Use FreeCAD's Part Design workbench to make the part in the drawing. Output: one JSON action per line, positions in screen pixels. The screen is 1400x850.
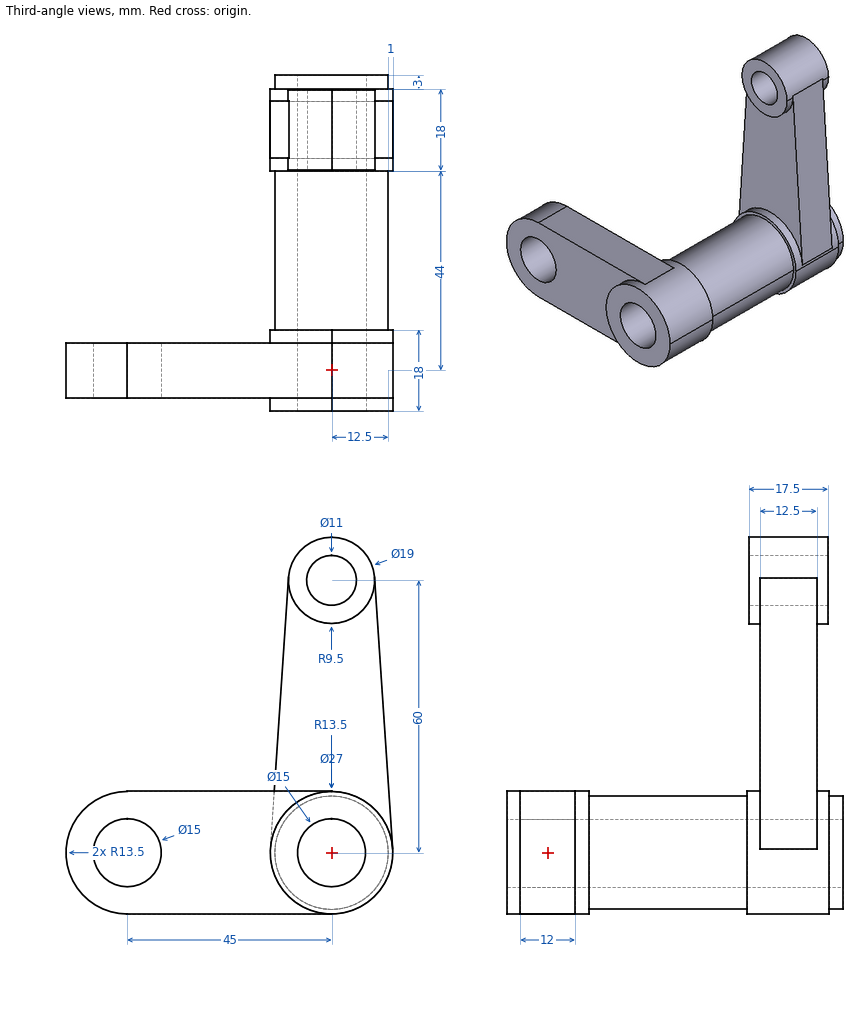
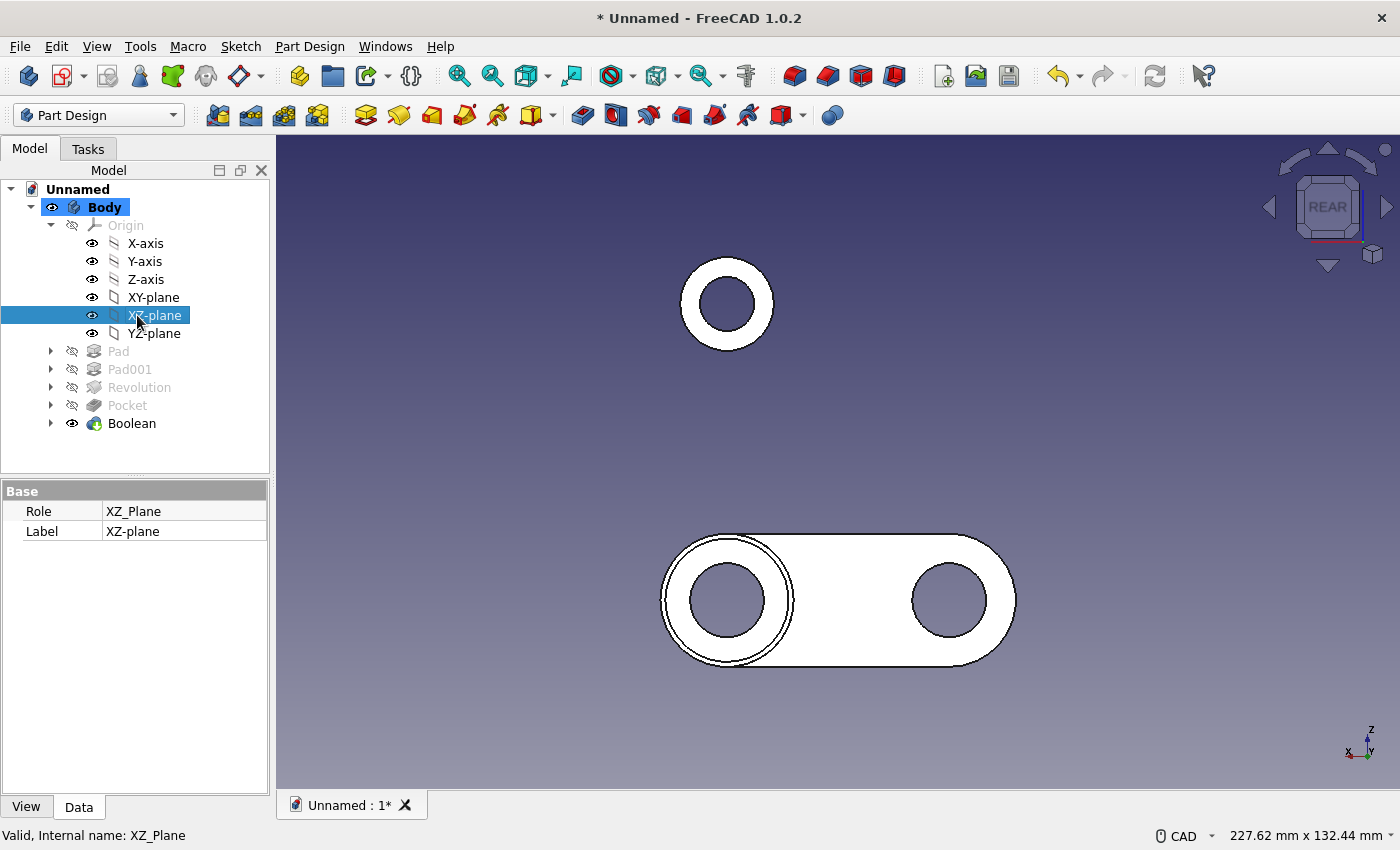
{"action": "left_click", "coordinate": [238, 76]}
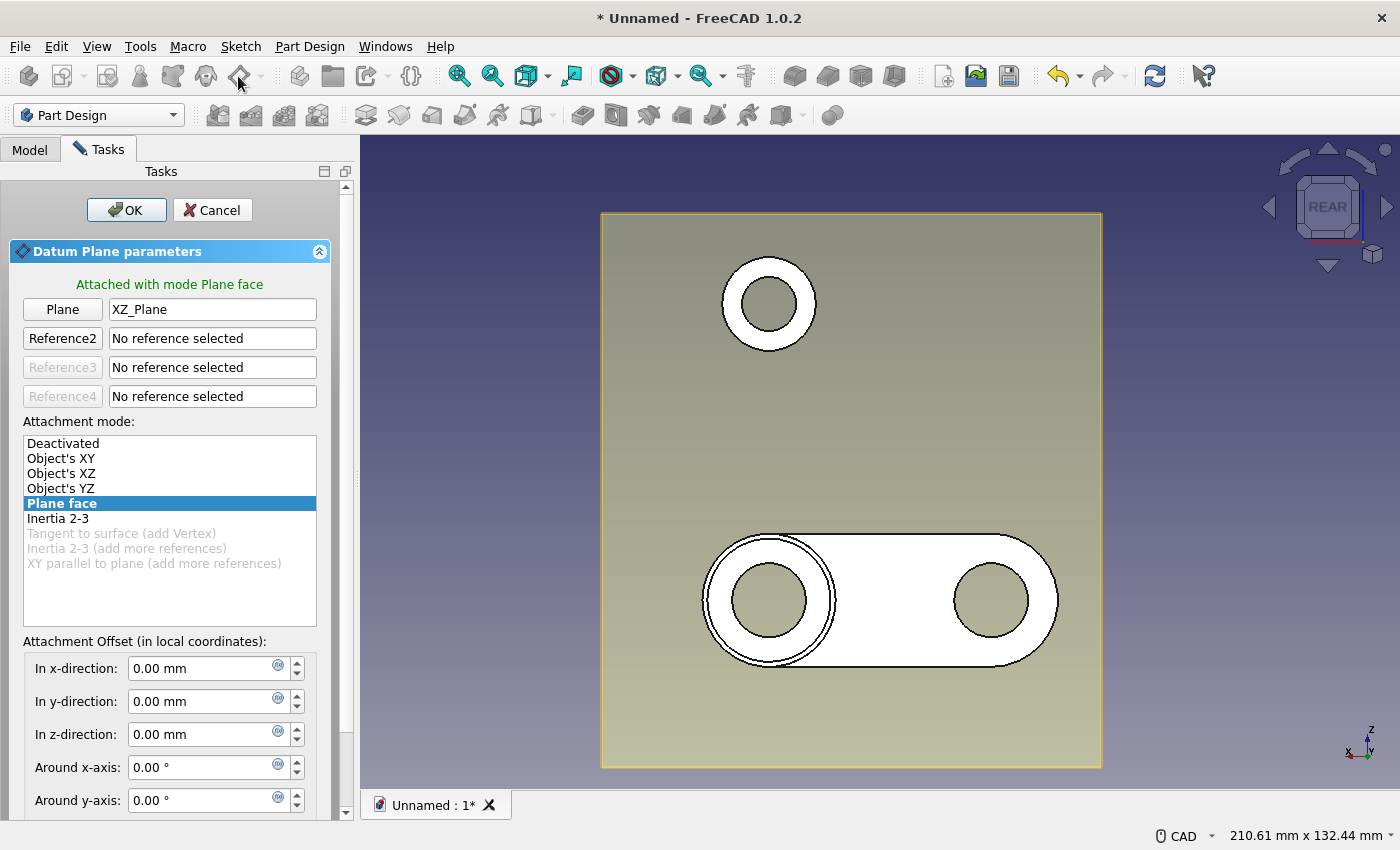
{"action": "triple_click", "coordinate": [210, 734]}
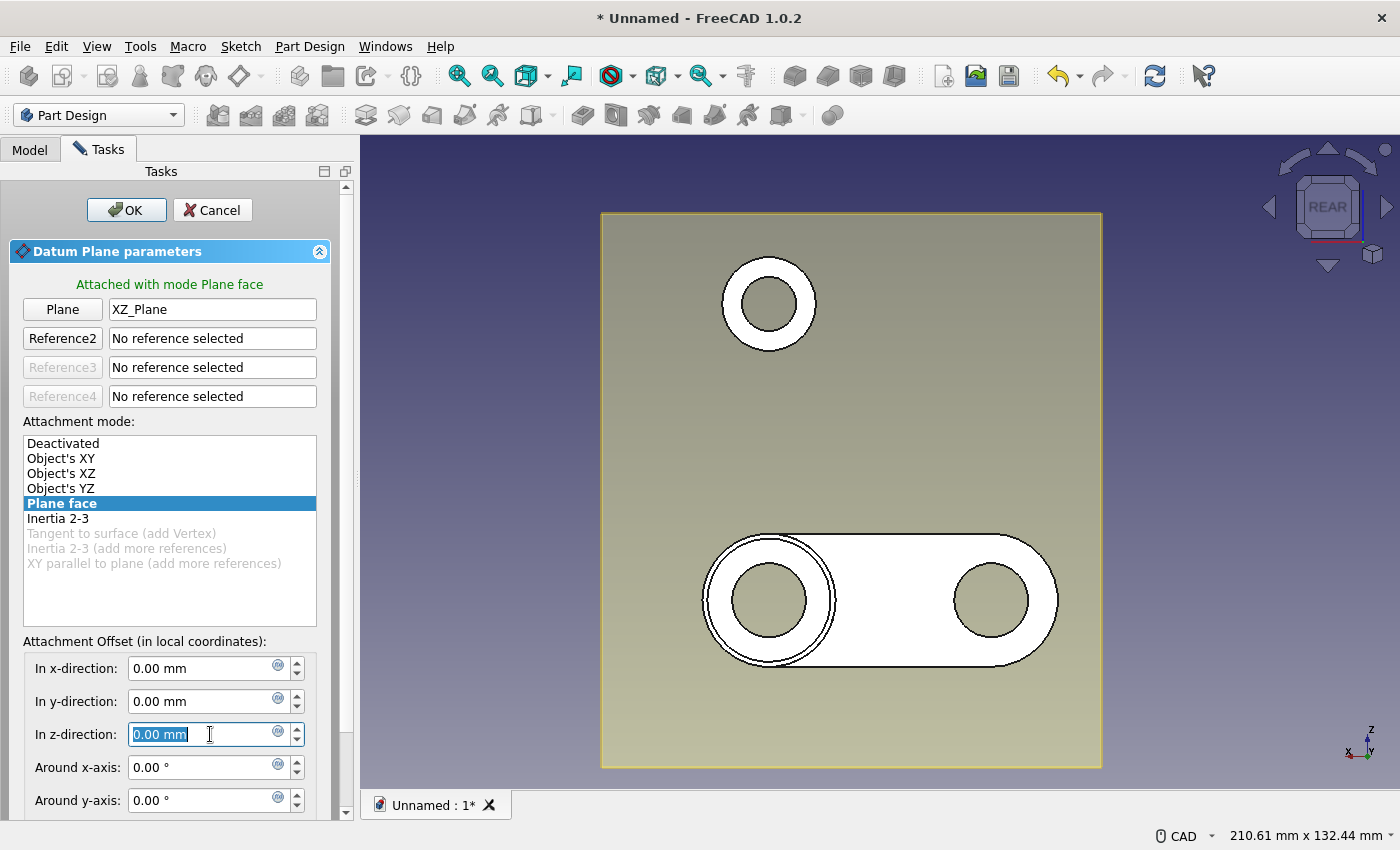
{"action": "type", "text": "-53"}
{"action": "key", "text": "Tab"}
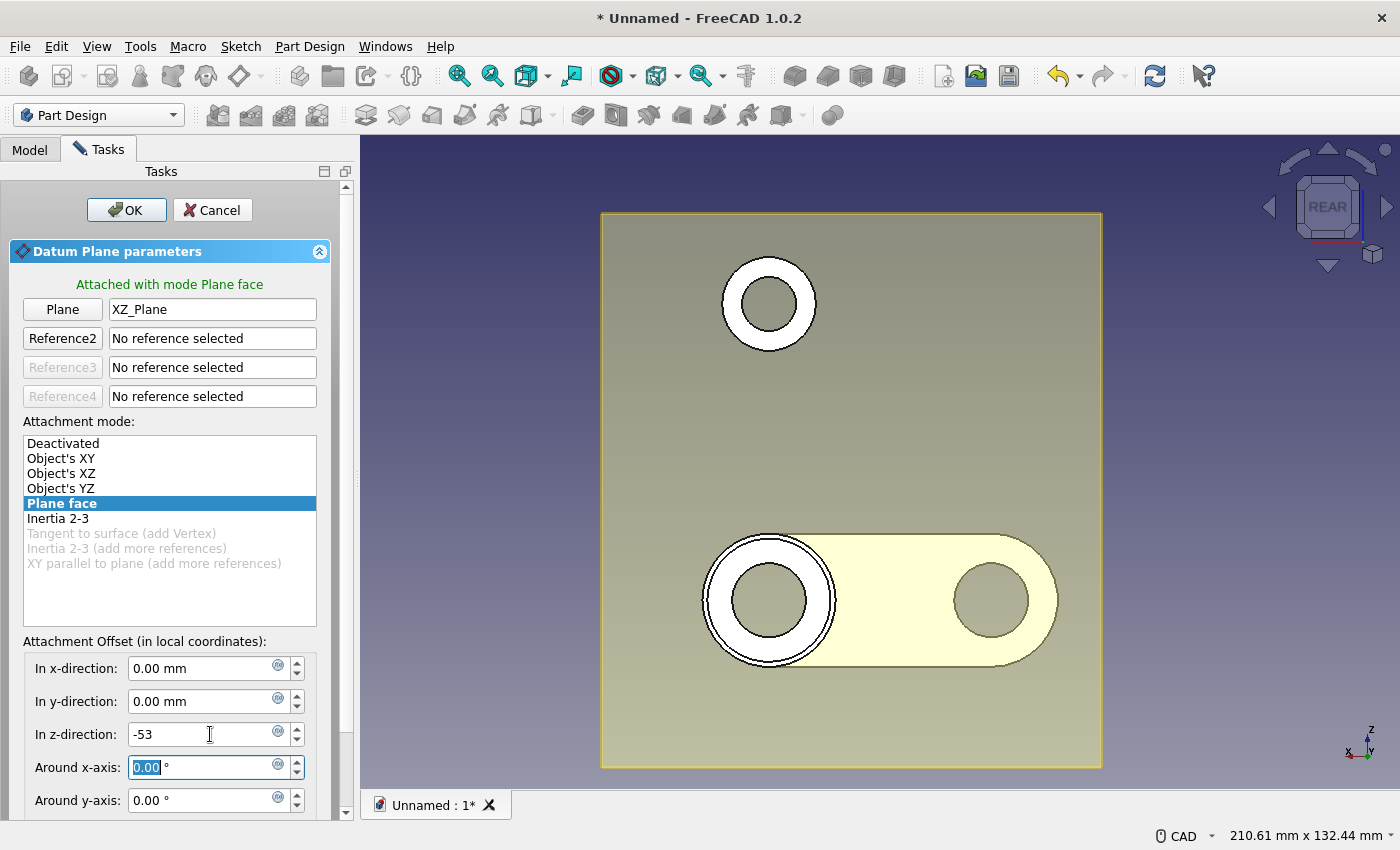
{"action": "left_click", "coordinate": [127, 210]}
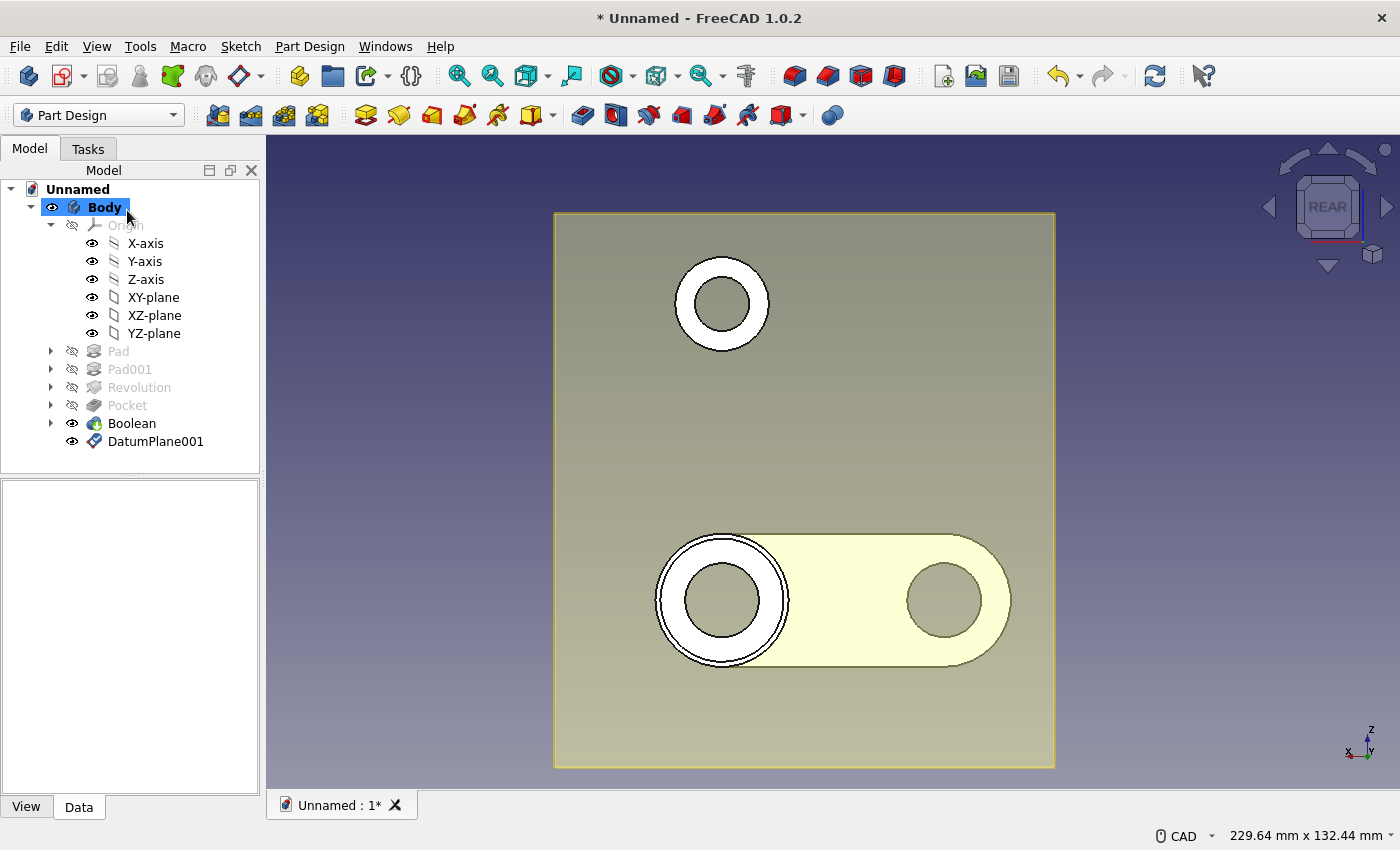
{"action": "left_click", "coordinate": [117, 441]}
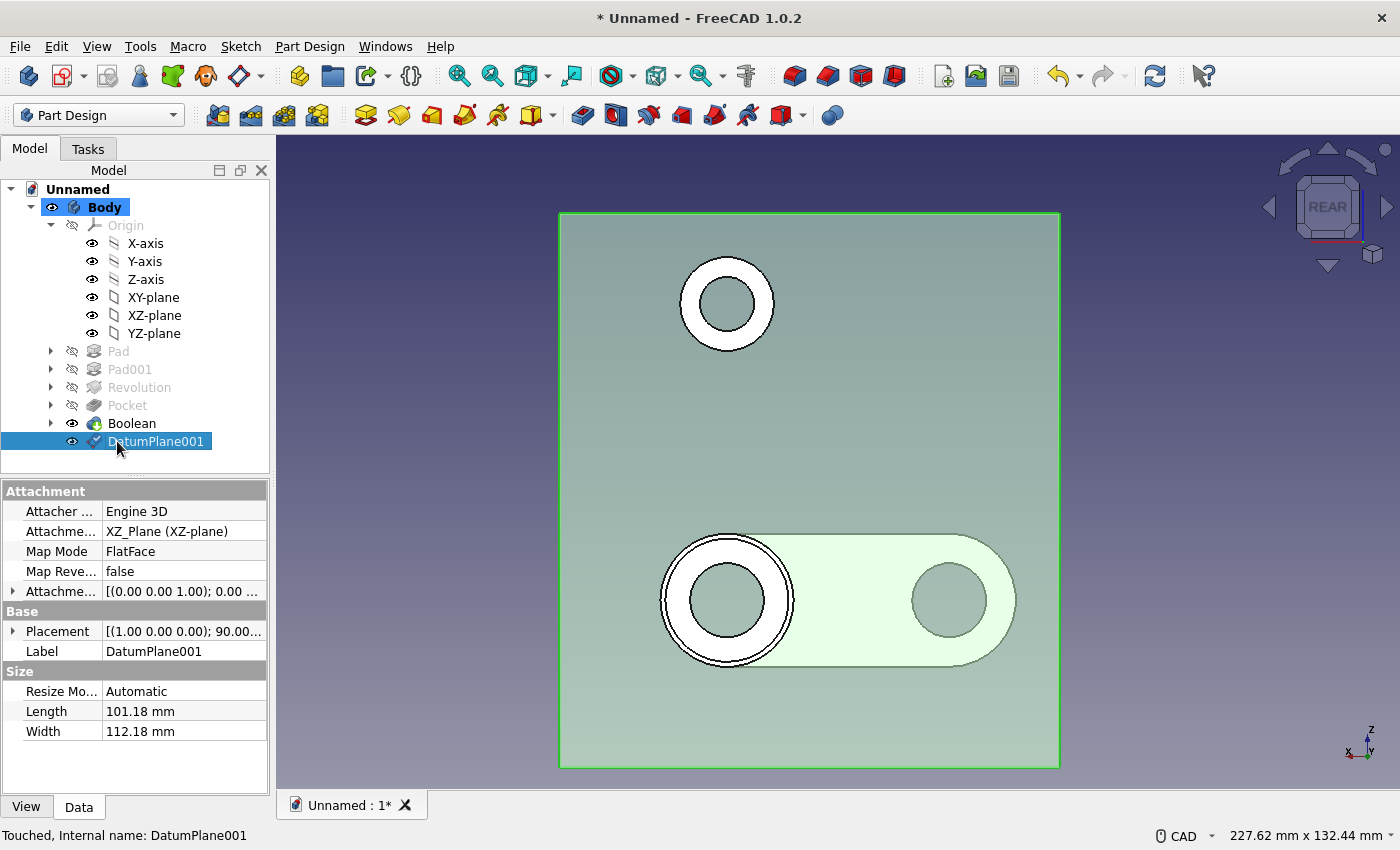
{"action": "left_click", "coordinate": [62, 76]}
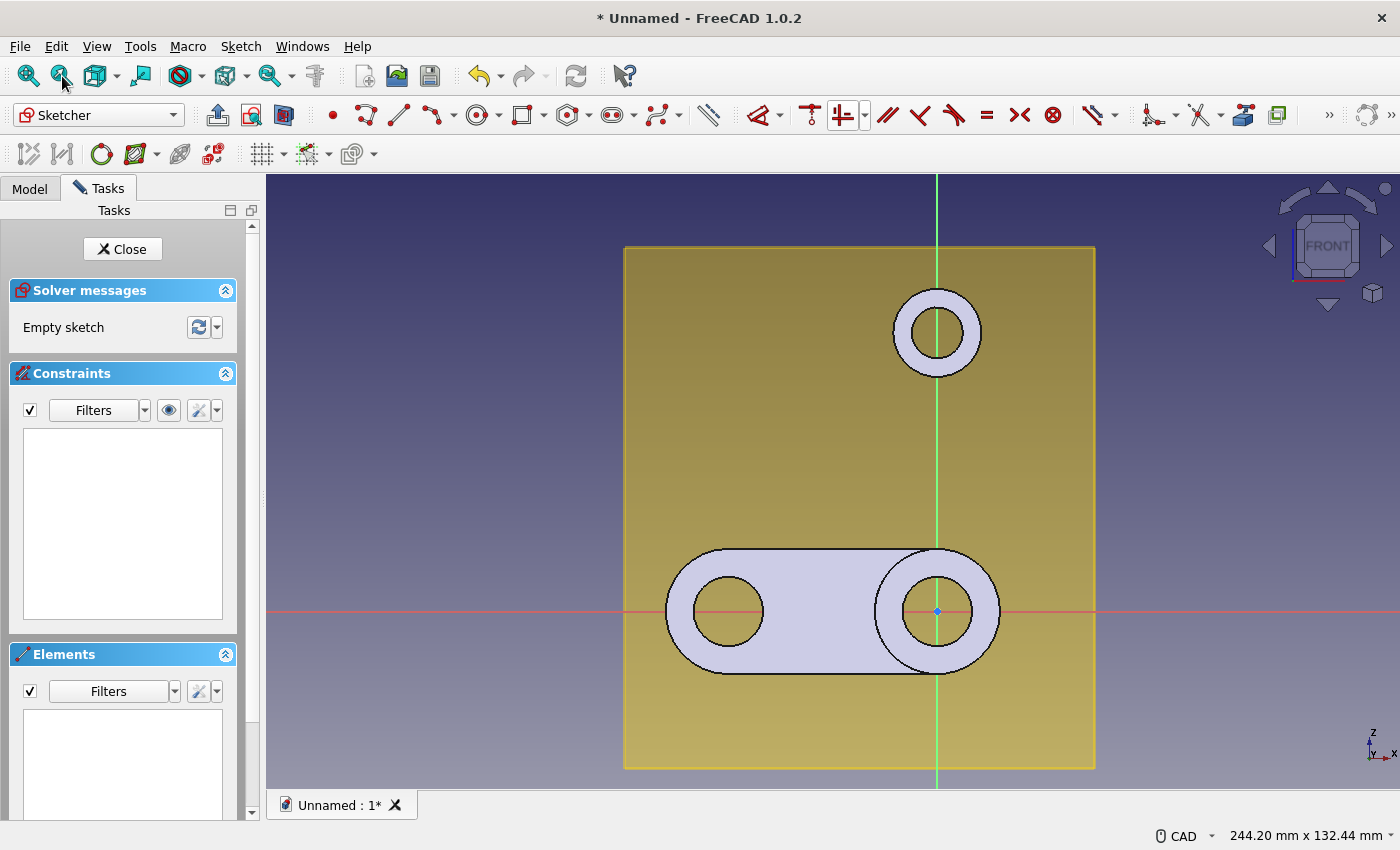
{"action": "key", "text": "q s"}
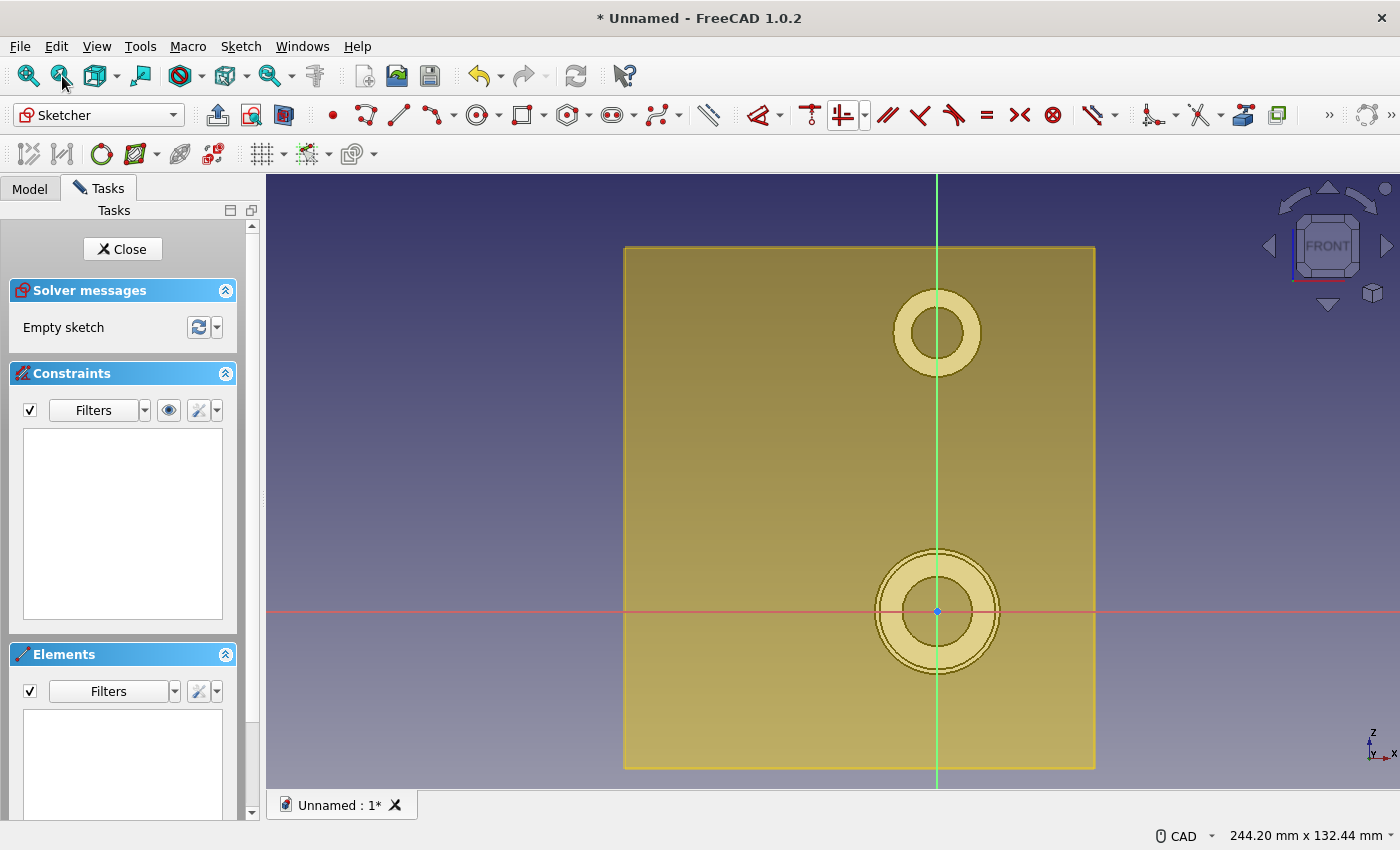
{"action": "scroll", "coordinate": [1235, 449], "scroll_direction": "up", "scroll_amount": 2}